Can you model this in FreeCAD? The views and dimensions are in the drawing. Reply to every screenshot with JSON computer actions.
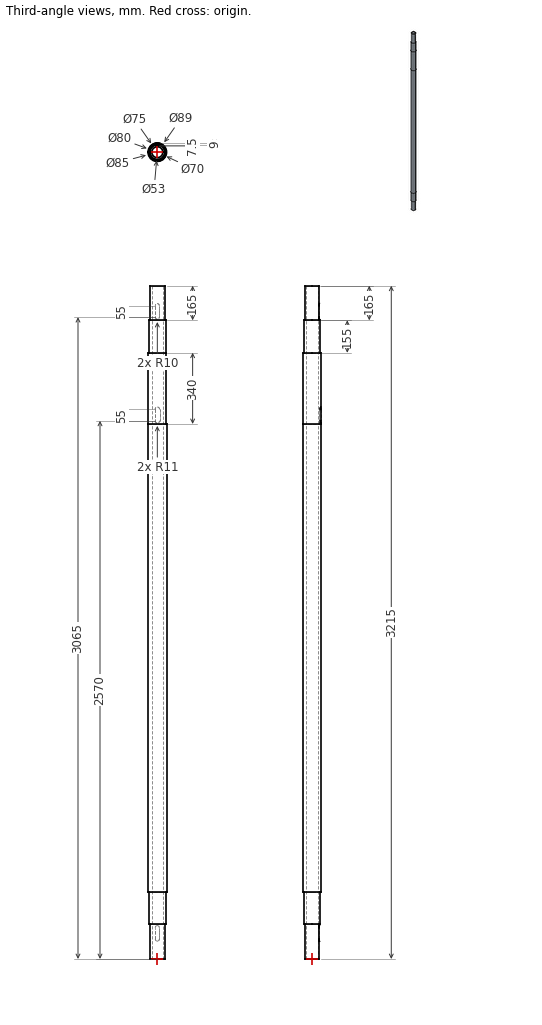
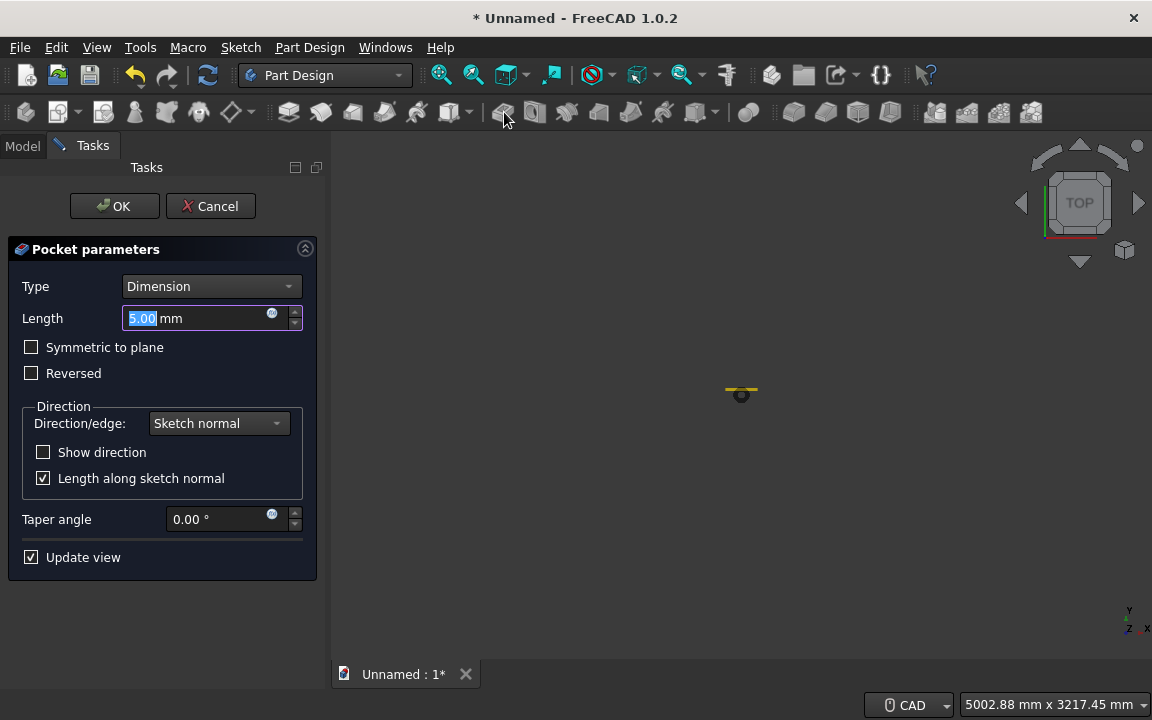
{"action": "type", "text": "7.5"}
{"action": "key", "text": "Tab"}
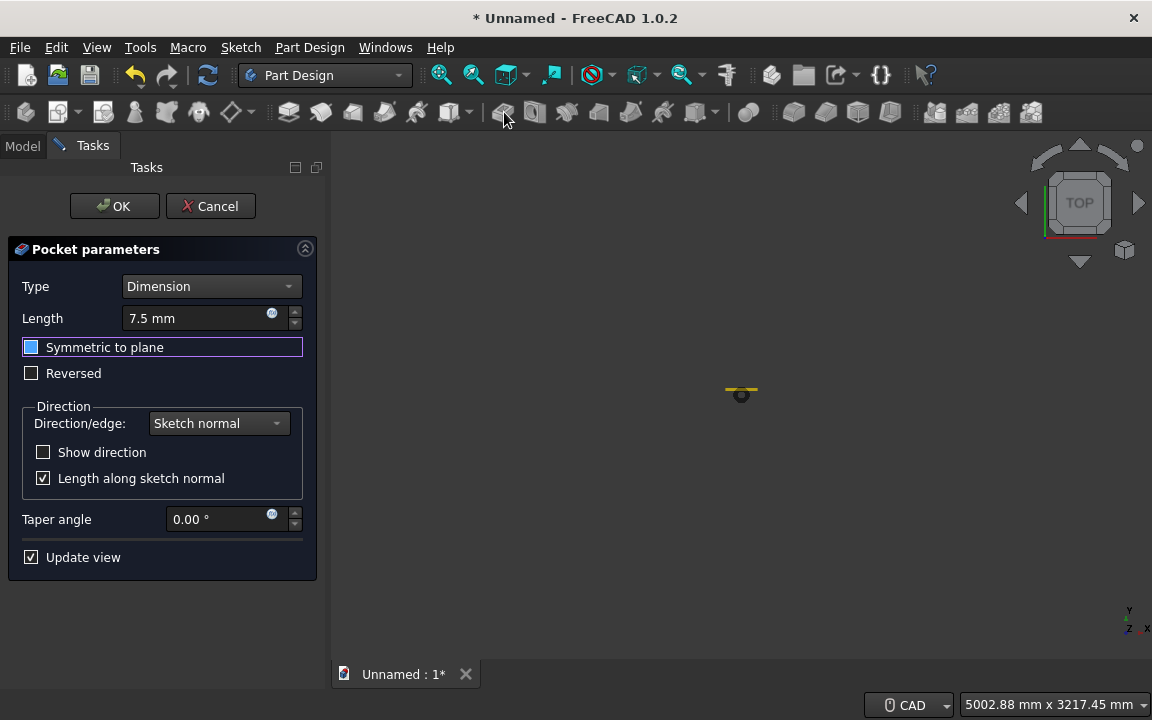
{"action": "left_click", "coordinate": [30, 373]}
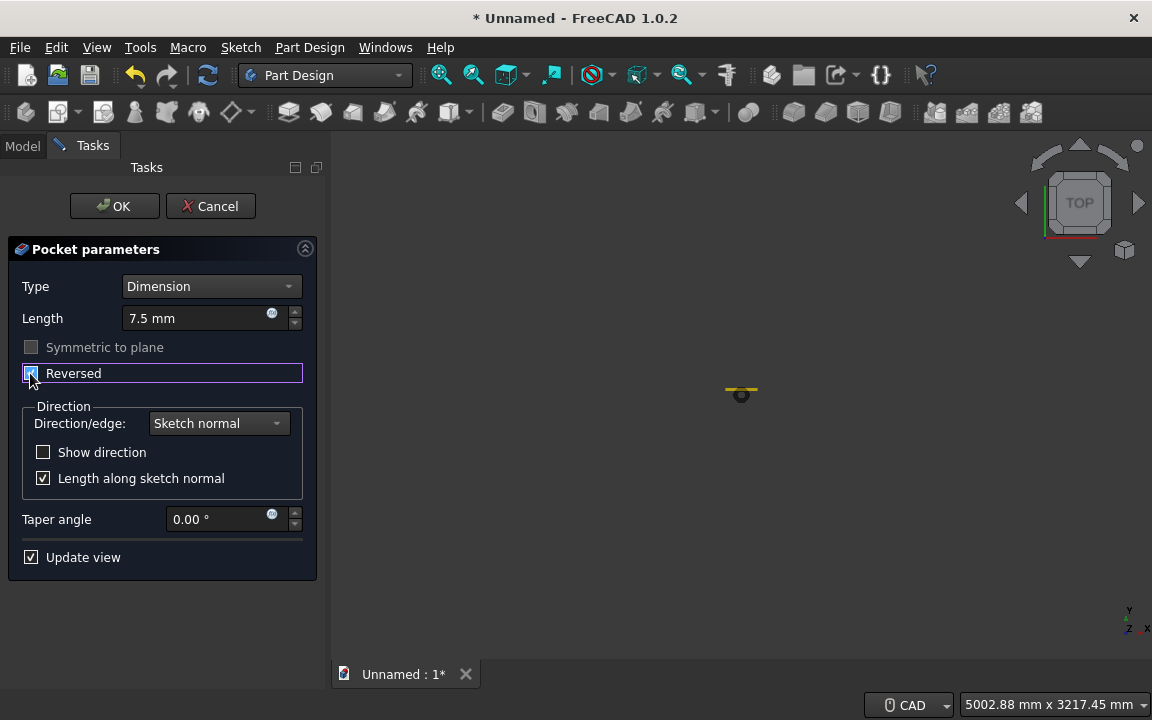
{"action": "left_click", "coordinate": [115, 206]}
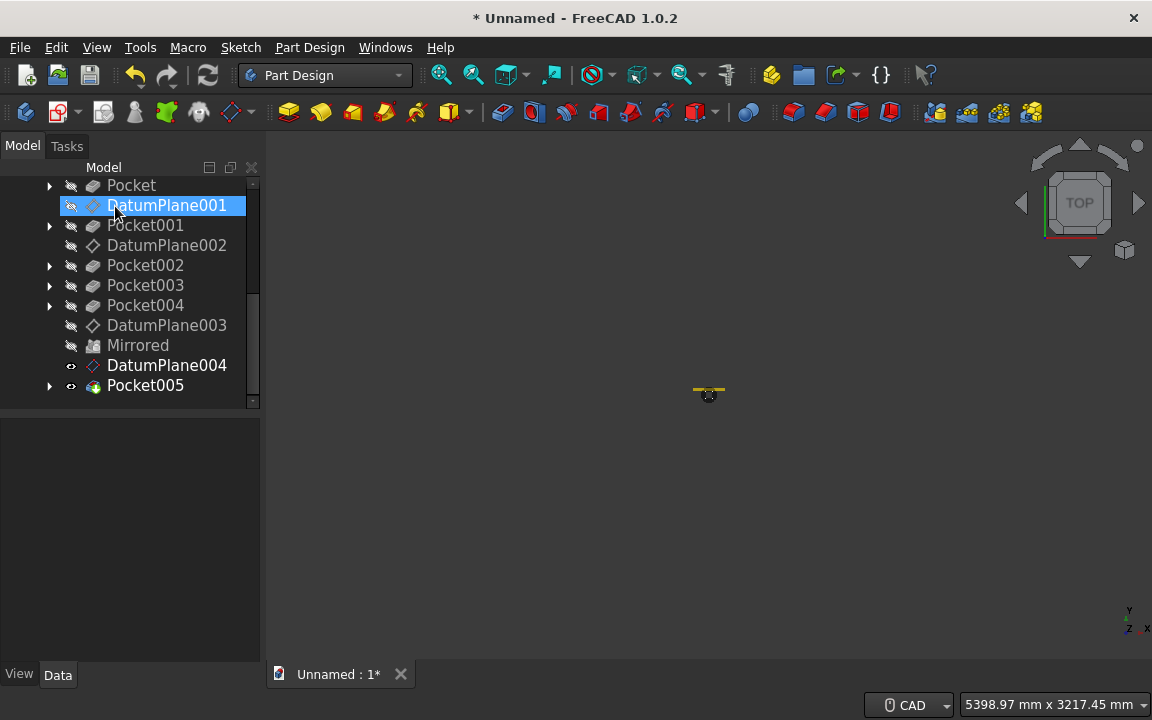
{"action": "left_click", "coordinate": [116, 366]}
{"action": "key", "text": "space"}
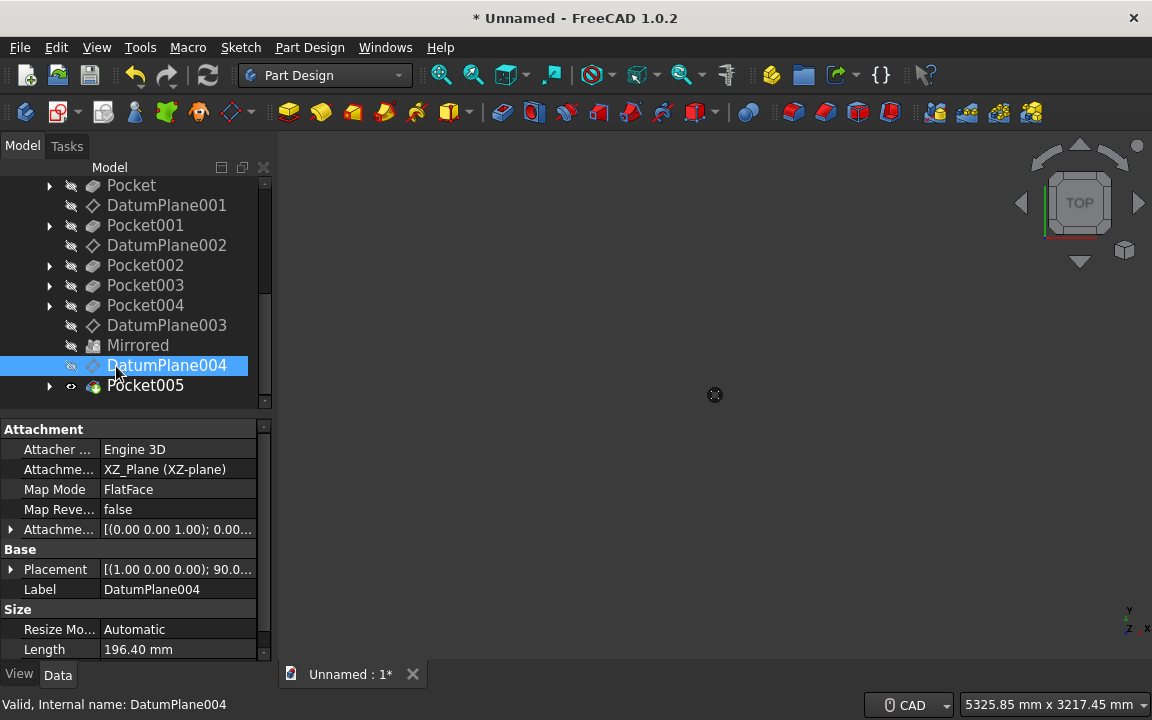
{"action": "left_click", "coordinate": [442, 76]}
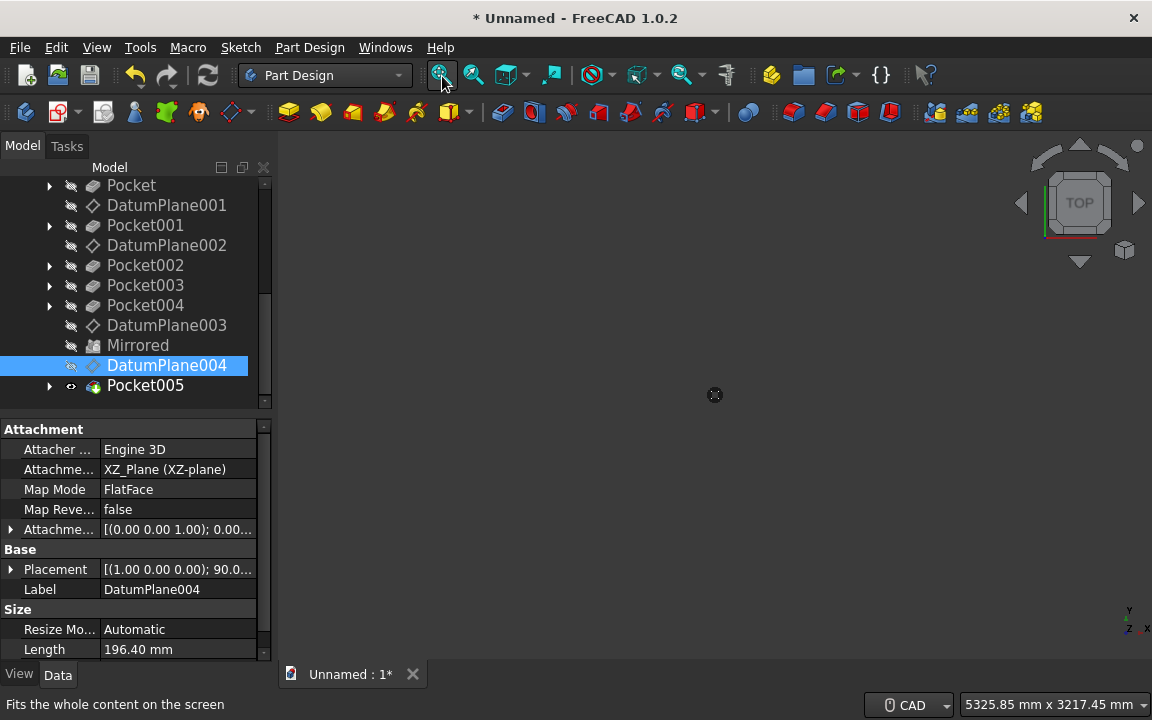
{"action": "scroll", "coordinate": [140, 281], "scroll_direction": "down", "scroll_amount": 3}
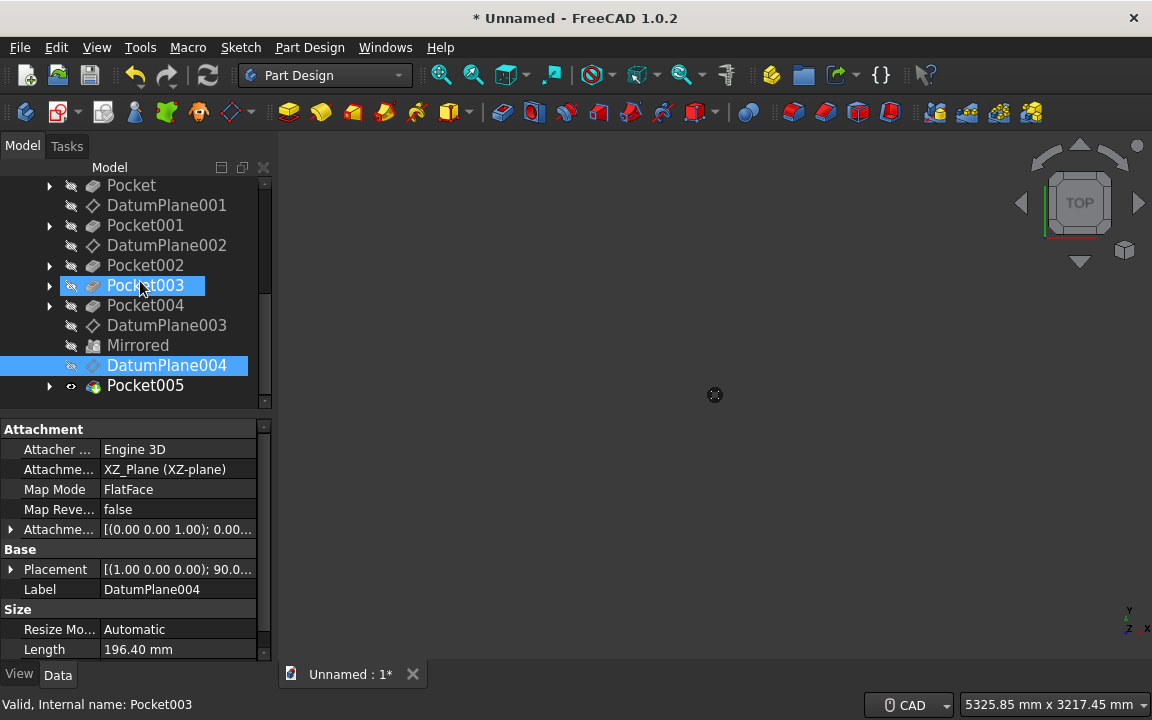
{"action": "scroll", "coordinate": [140, 281], "scroll_direction": "up", "scroll_amount": 15}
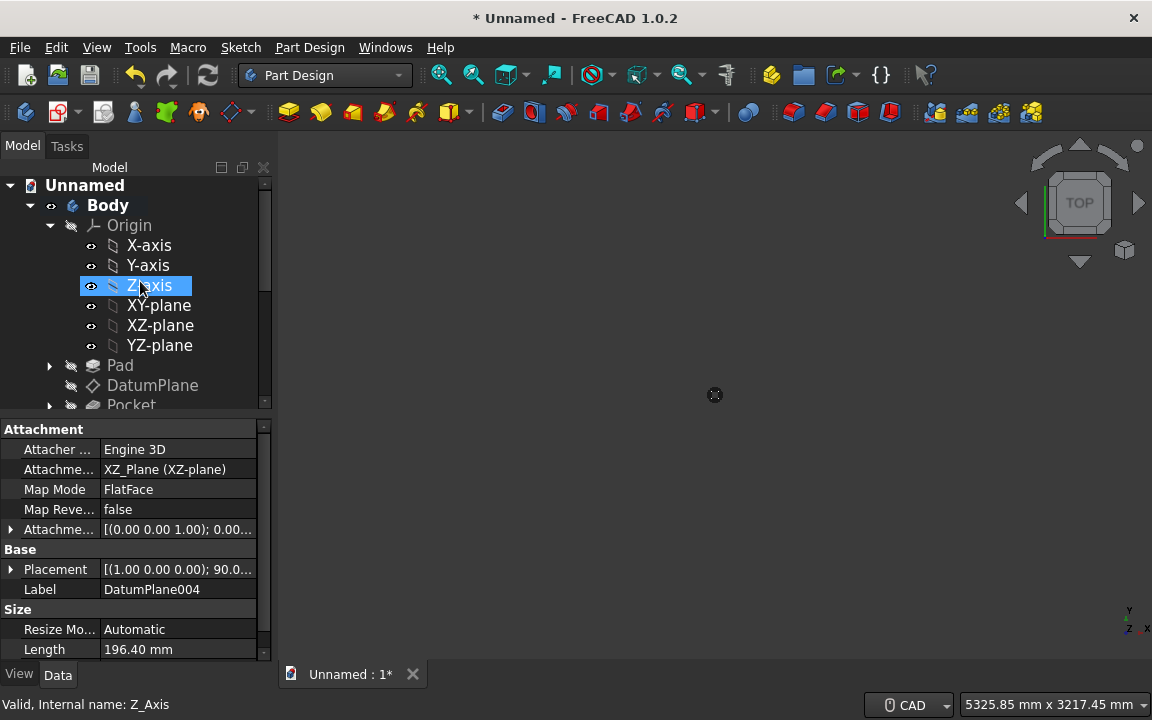
{"action": "left_click", "coordinate": [136, 306]}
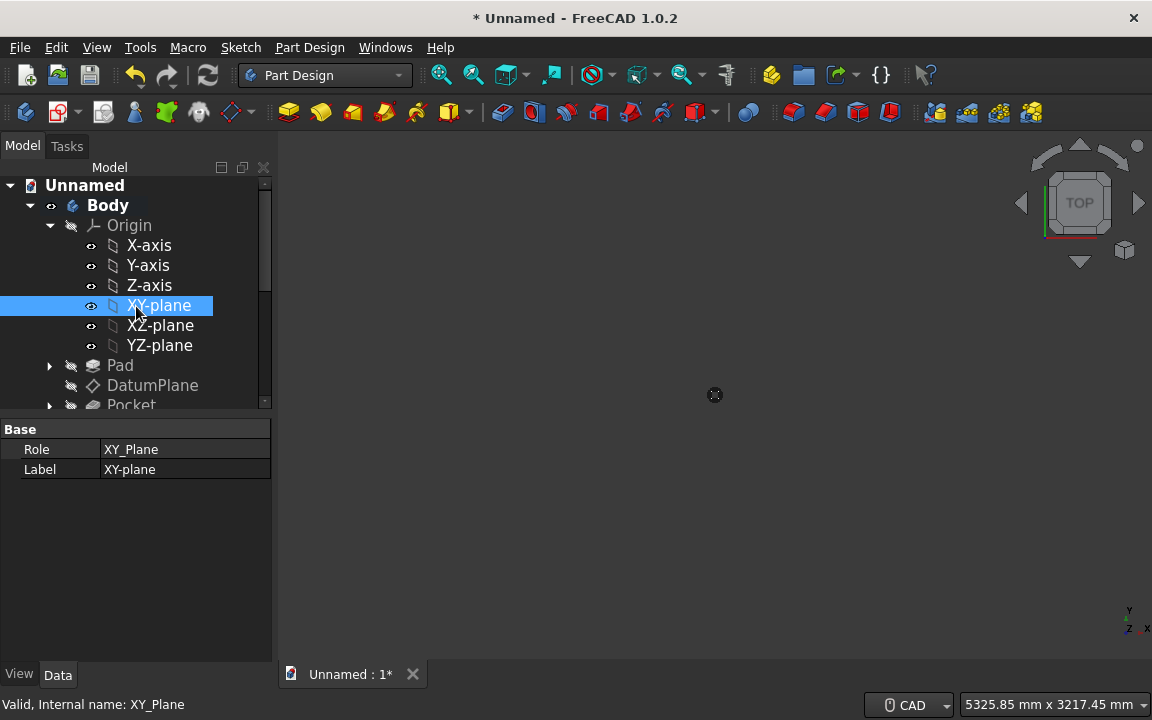
{"action": "left_click", "coordinate": [232, 112]}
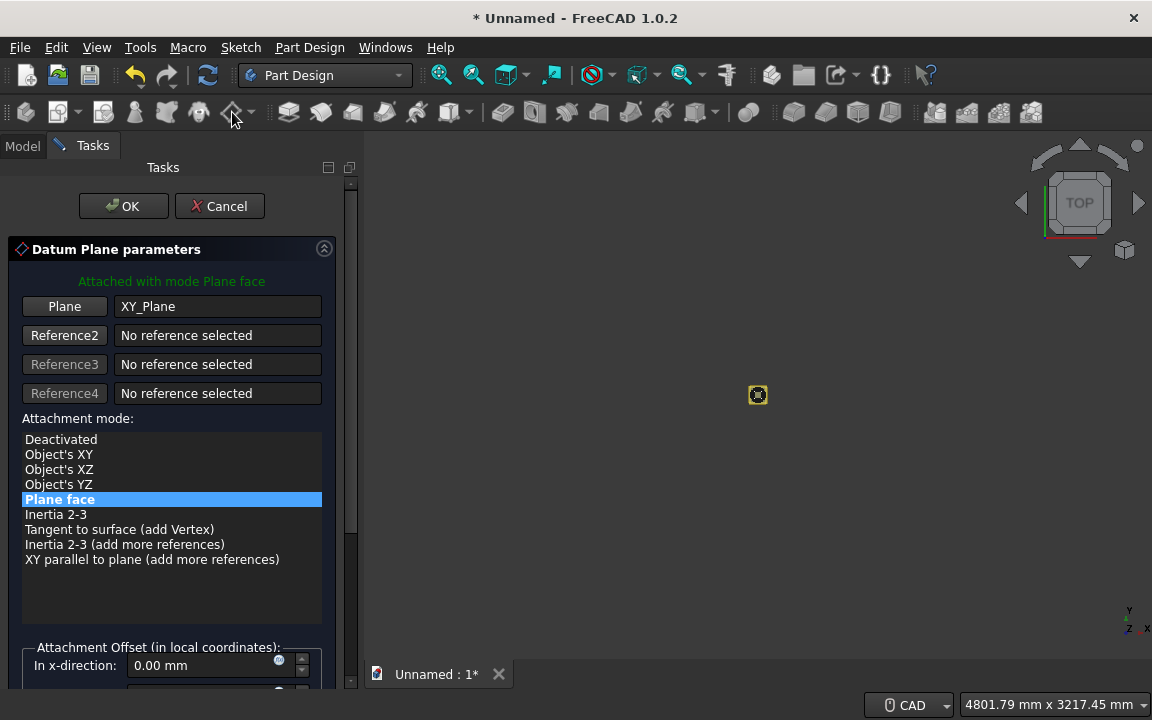
{"action": "scroll", "coordinate": [351, 432], "scroll_direction": "down", "scroll_amount": 2}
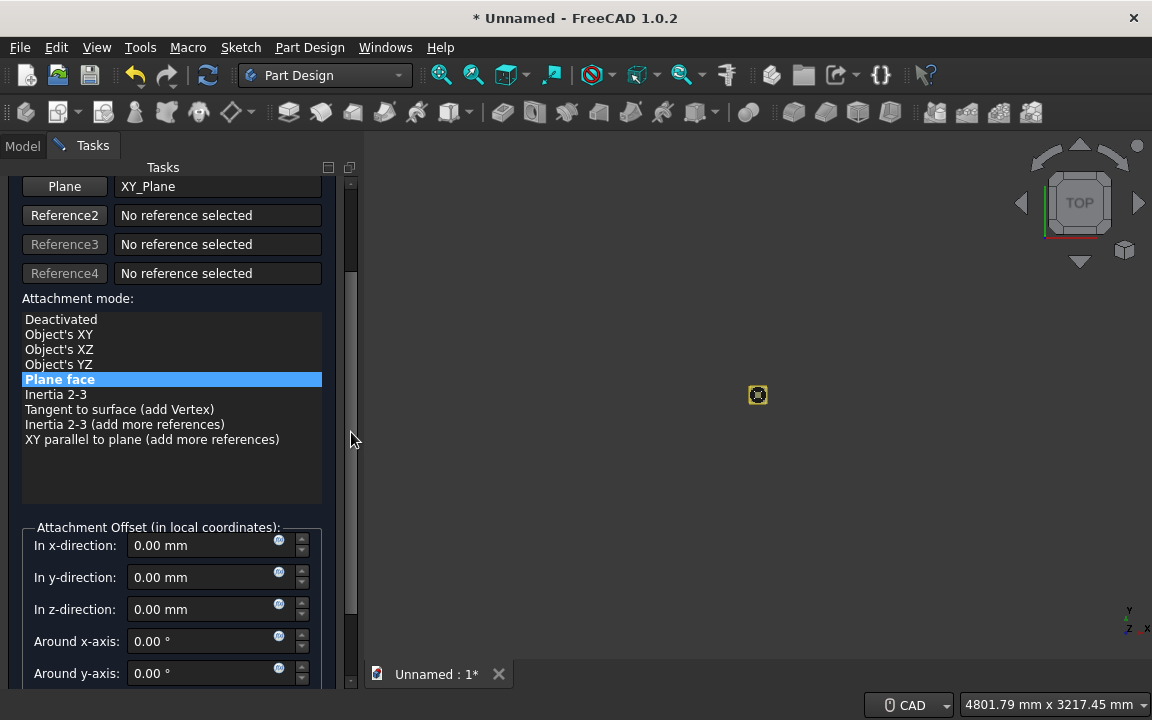
{"action": "triple_click", "coordinate": [210, 609]}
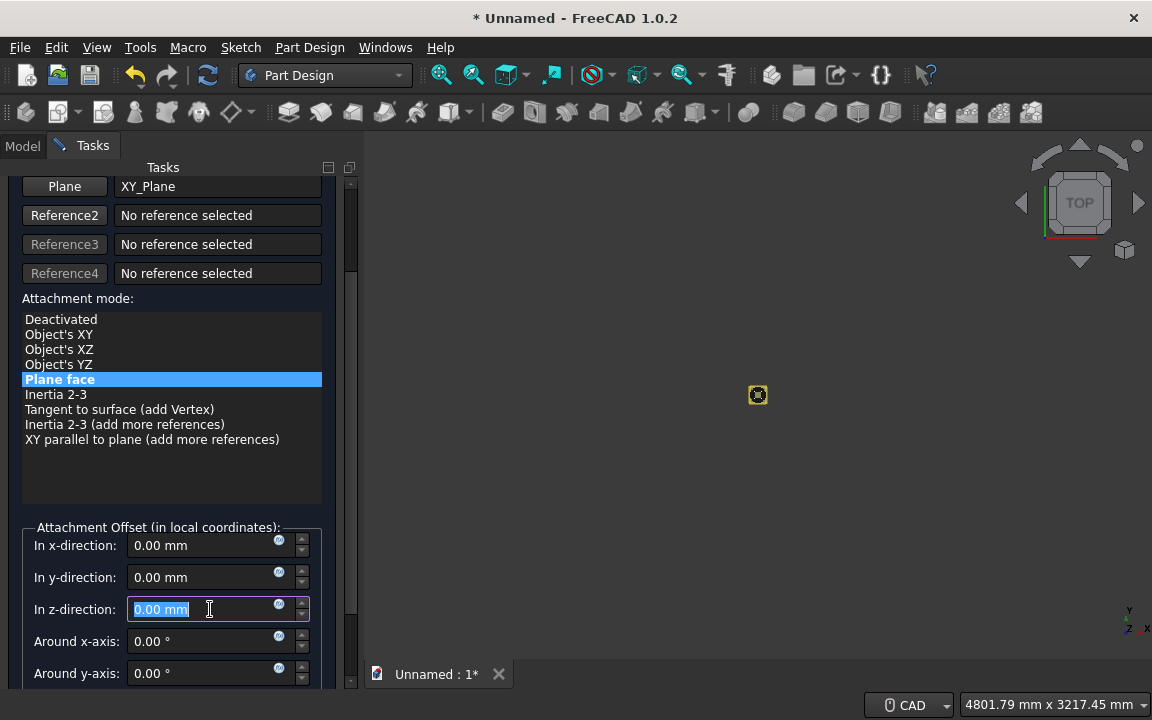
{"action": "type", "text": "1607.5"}
{"action": "key", "text": "Tab"}